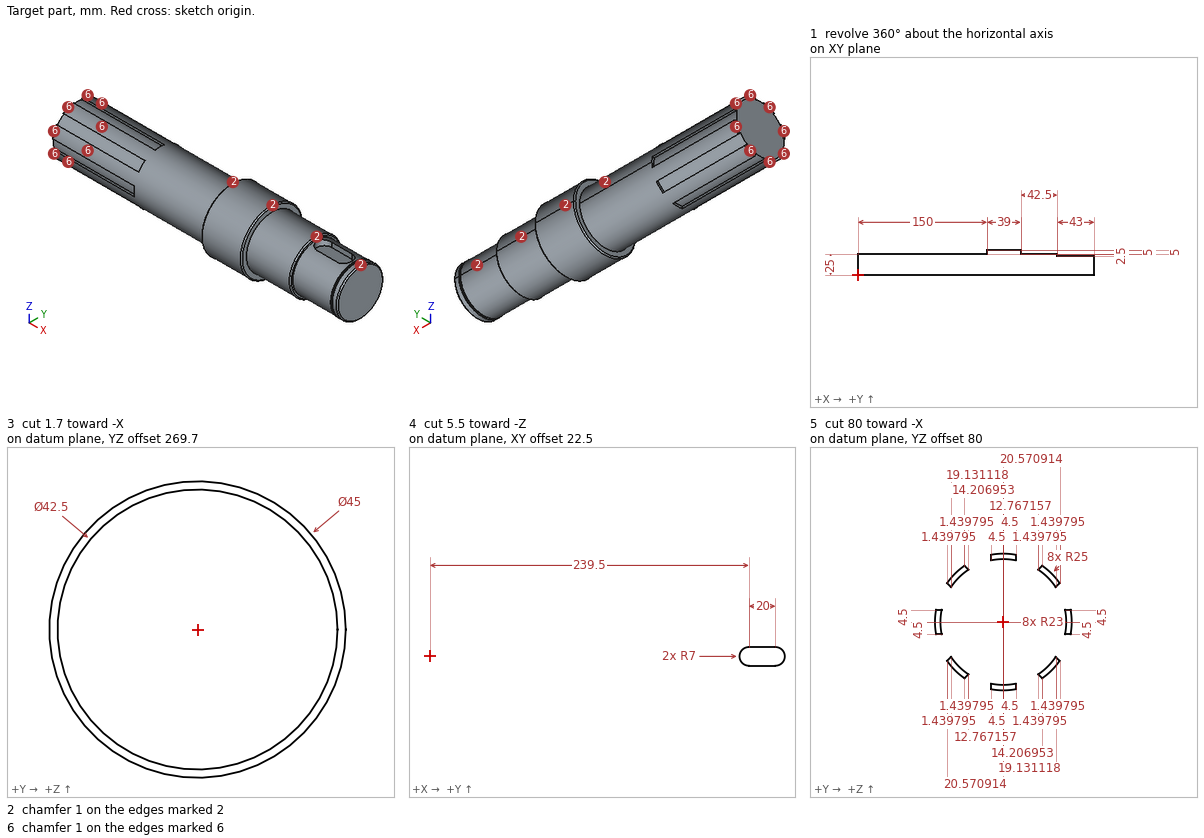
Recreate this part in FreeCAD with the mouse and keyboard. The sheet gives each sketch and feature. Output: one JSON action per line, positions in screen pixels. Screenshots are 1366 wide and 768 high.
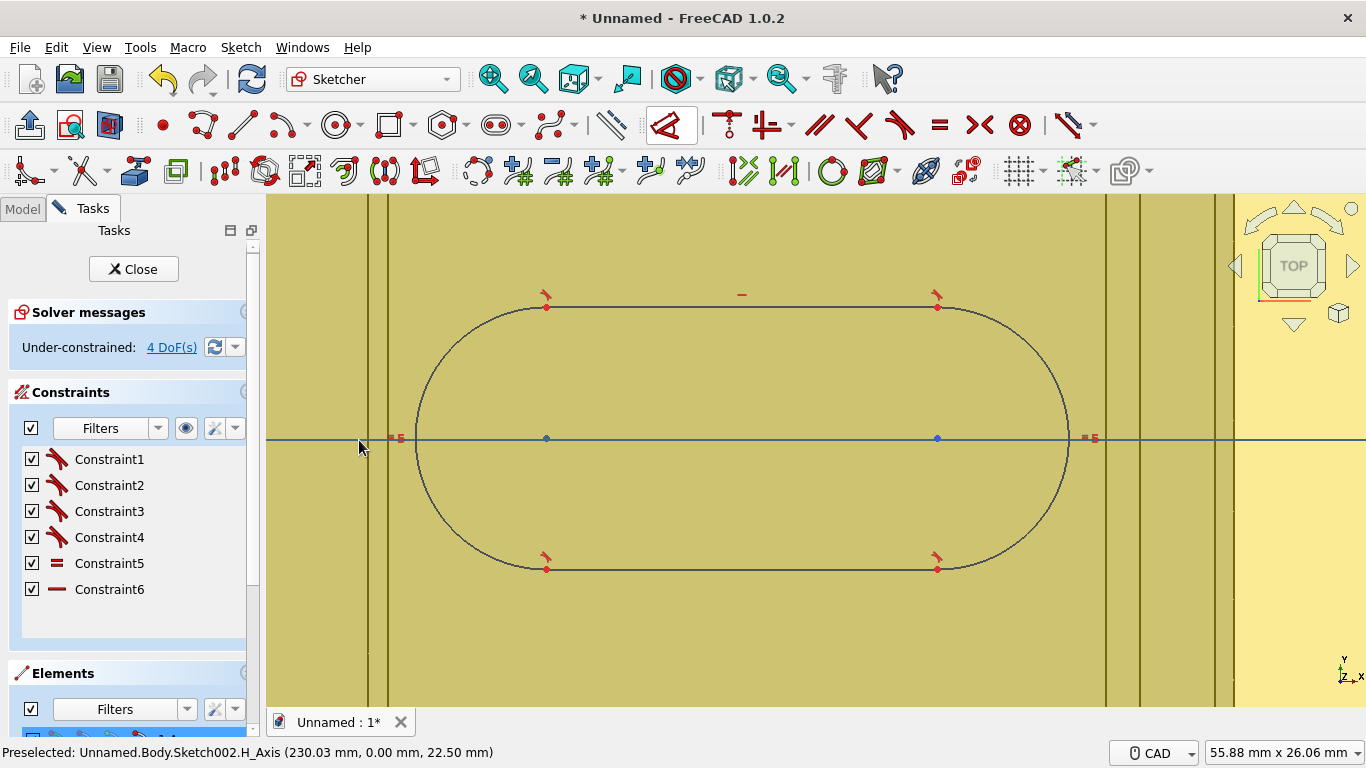
{"action": "left_click", "coordinate": [728, 126]}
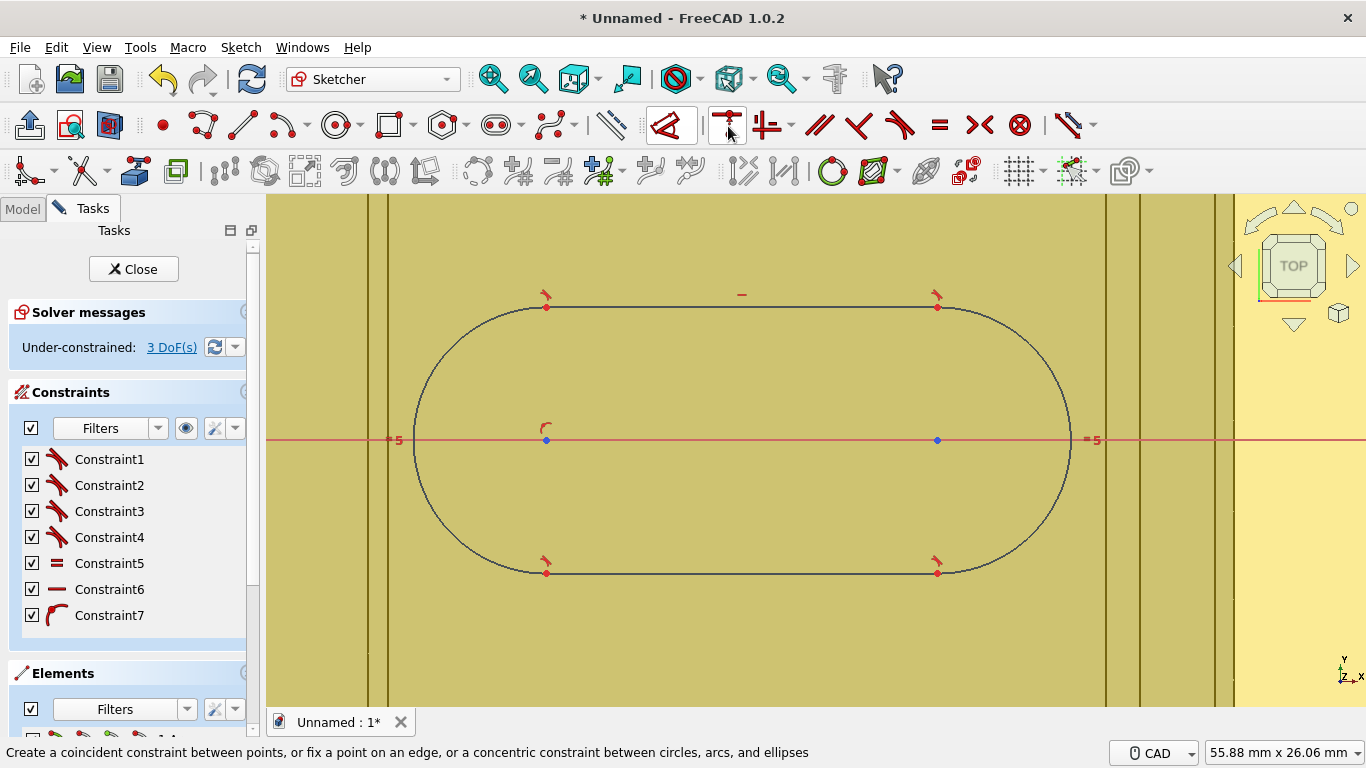
{"action": "left_click", "coordinate": [439, 362]}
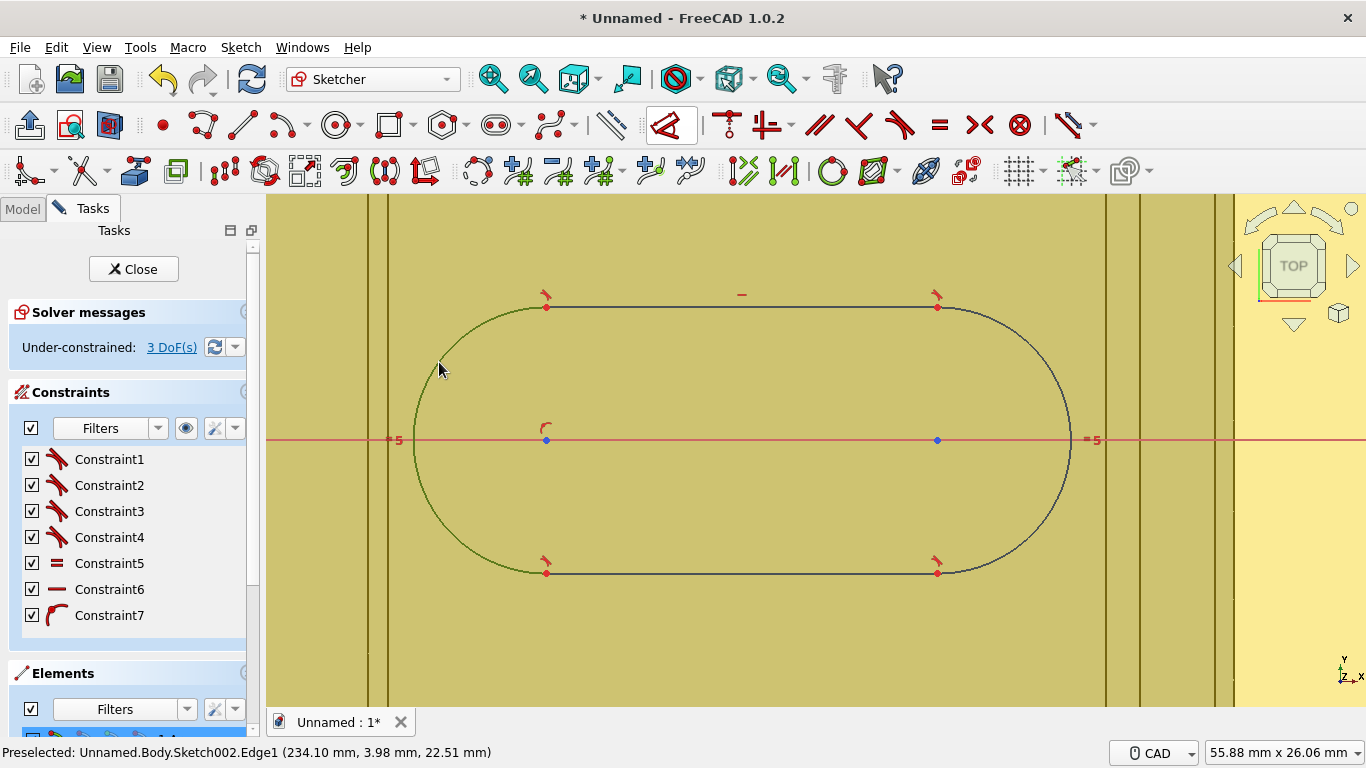
{"action": "key", "text": "k r"}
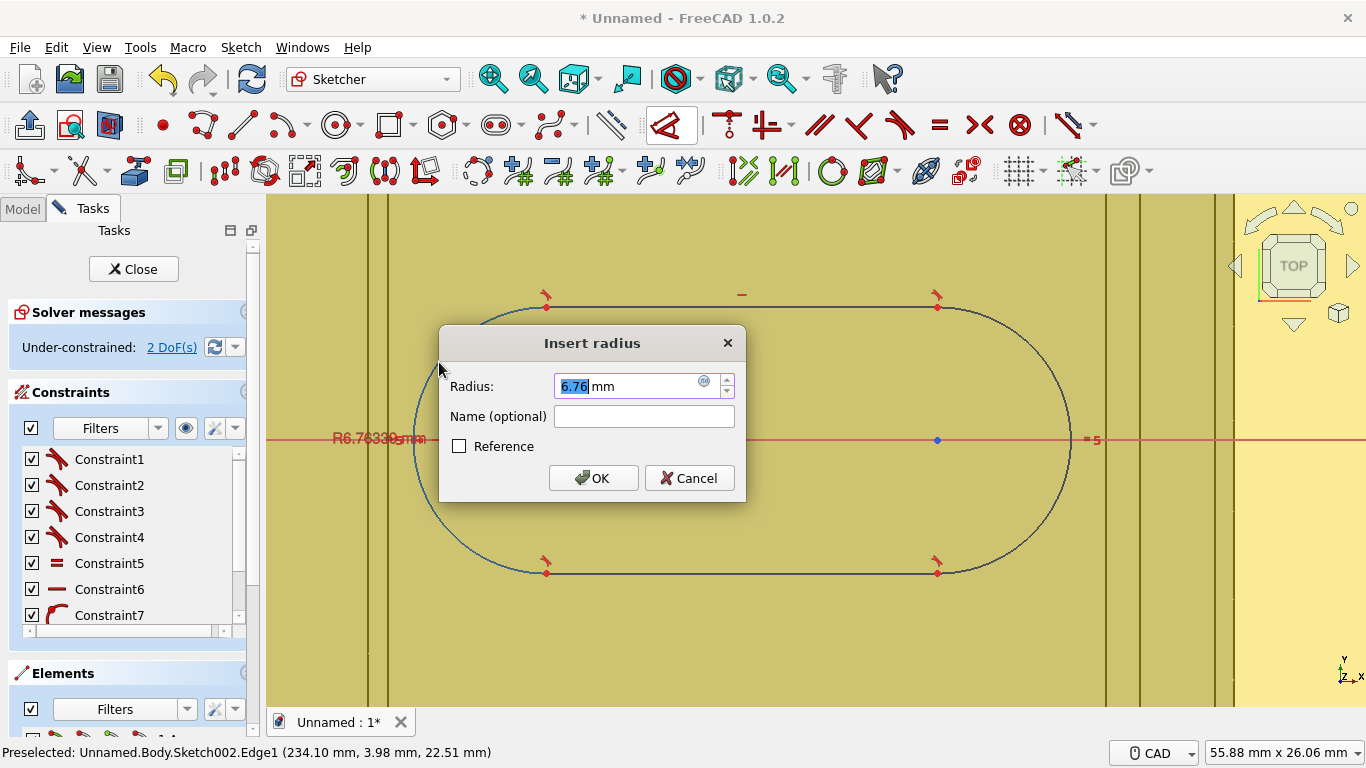
{"action": "type", "text": "7"}
{"action": "key", "text": "Return"}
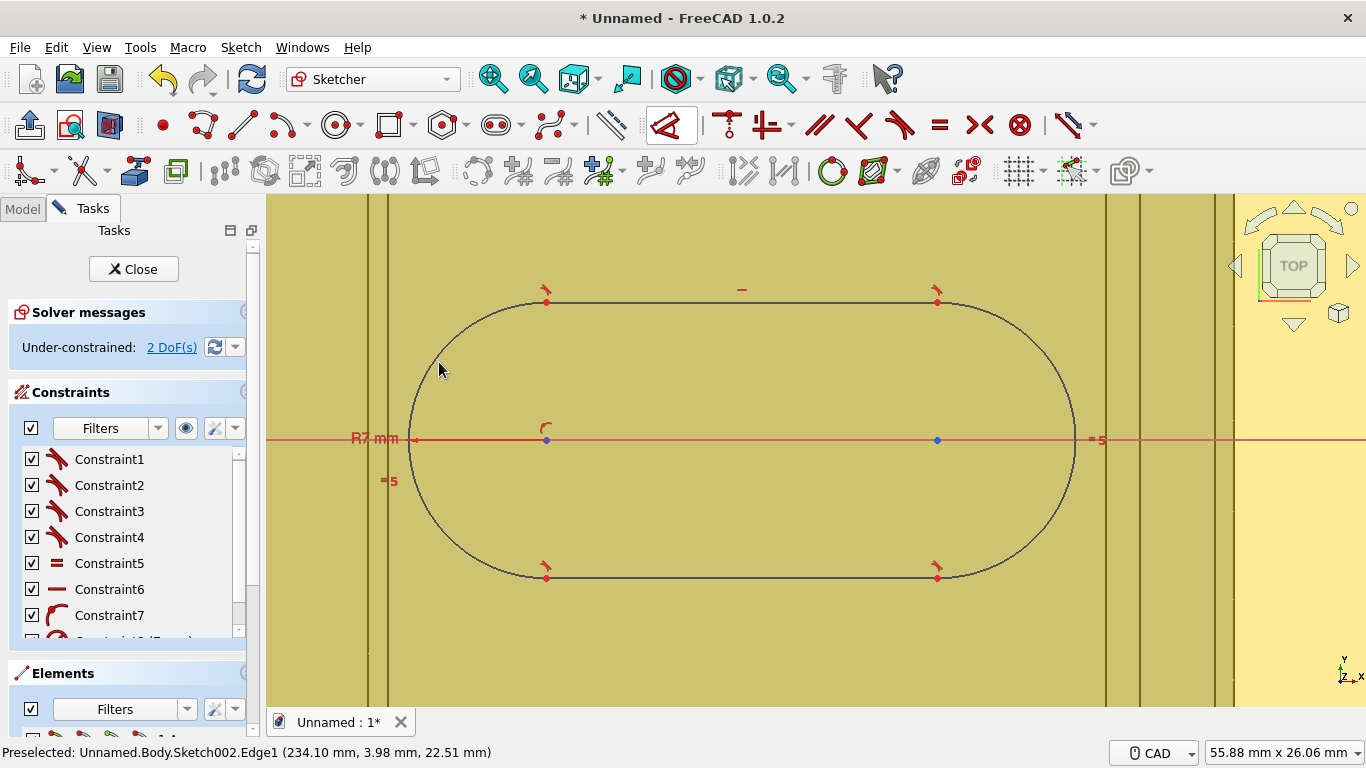
{"action": "left_click", "coordinate": [664, 303]}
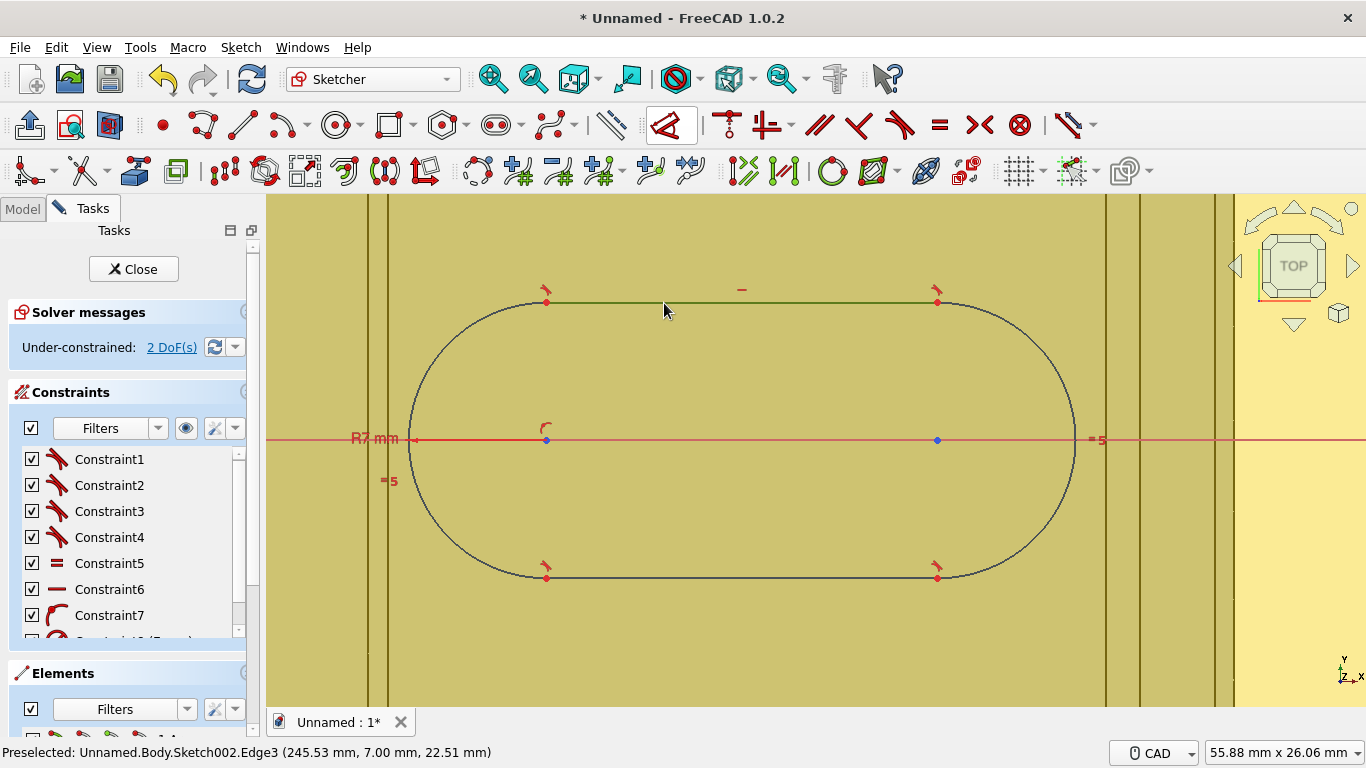
{"action": "key", "text": "l"}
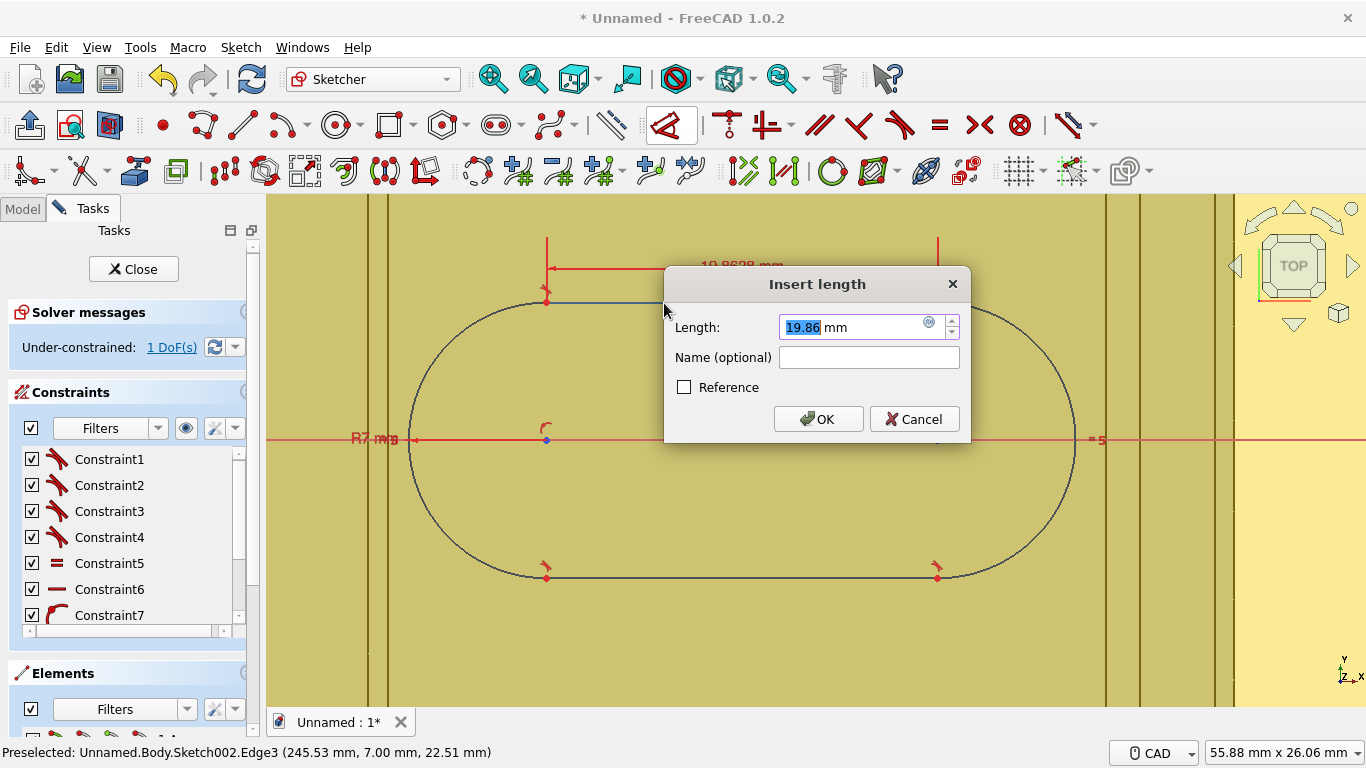
{"action": "type", "text": "20"}
{"action": "key", "text": "Return"}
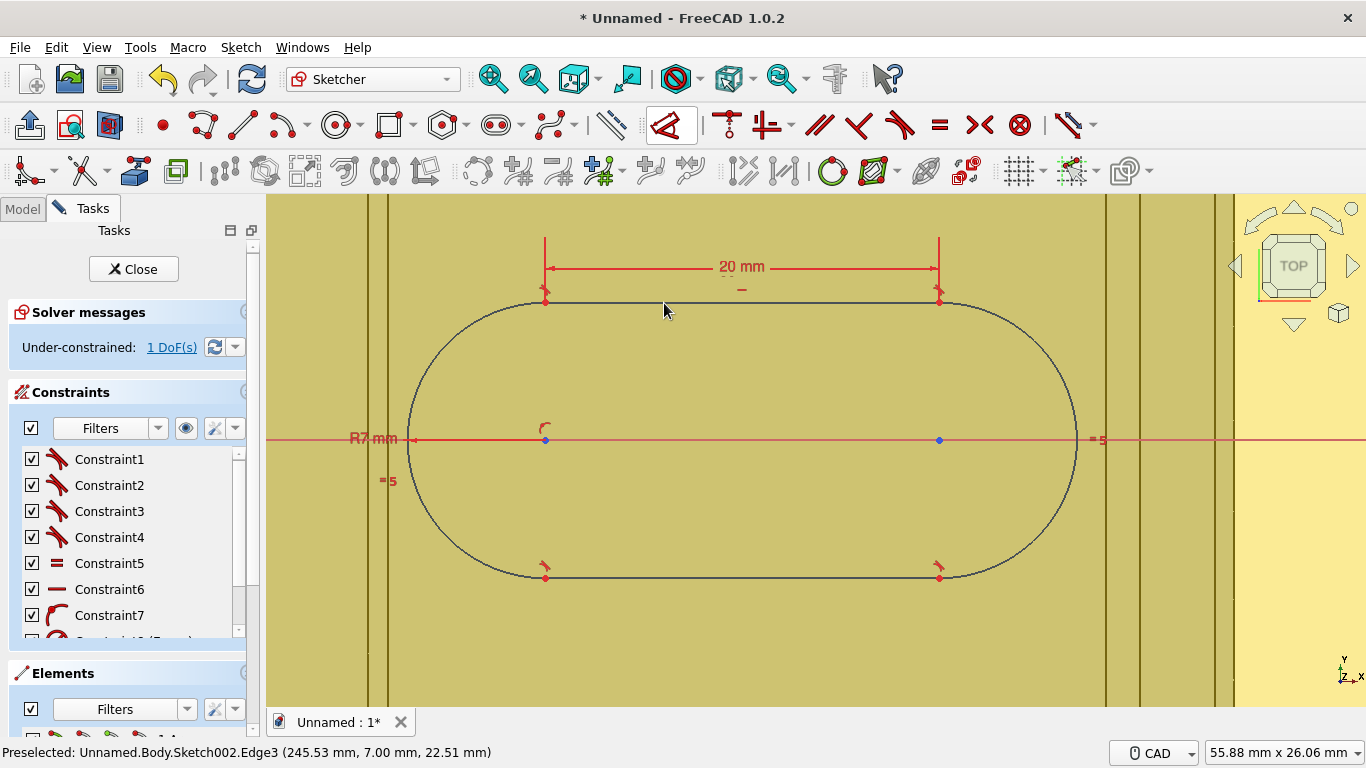
{"action": "left_click", "coordinate": [545, 303]}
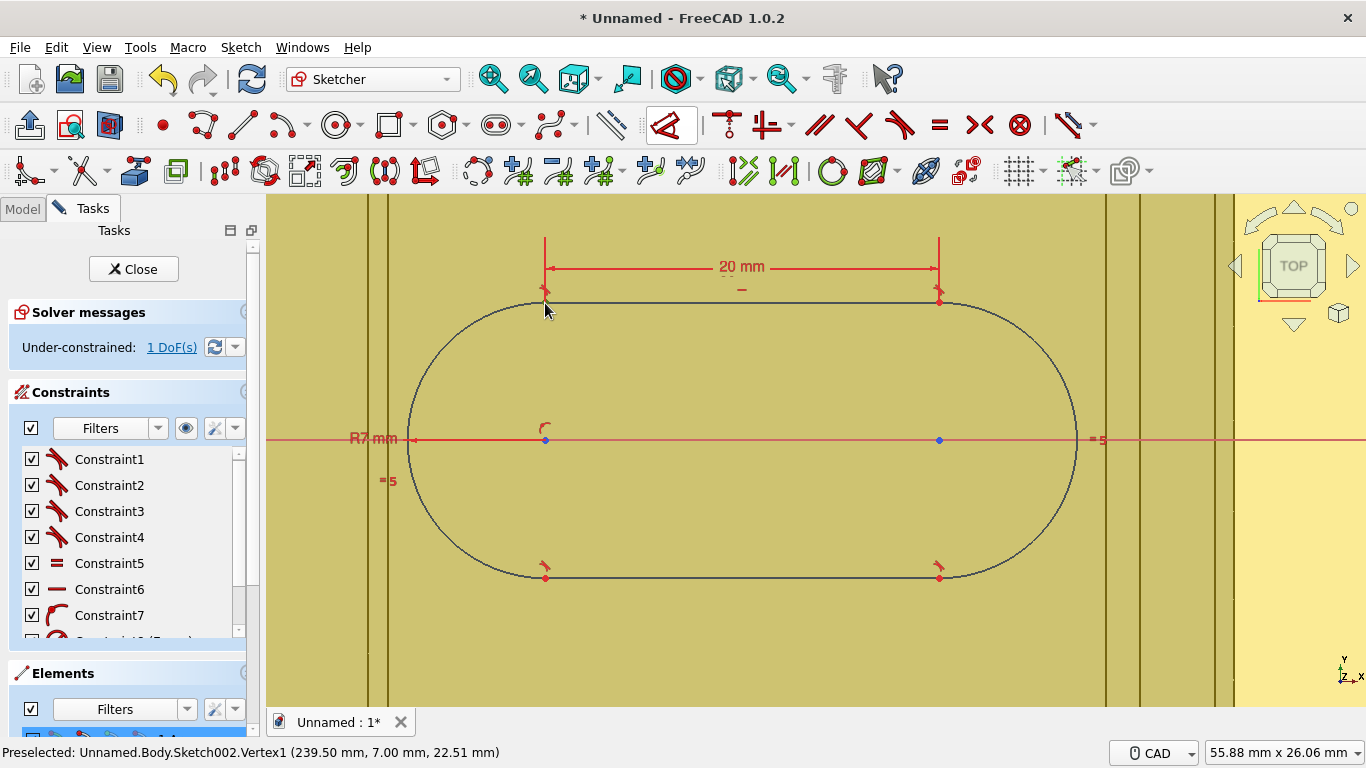
{"action": "key", "text": "l"}